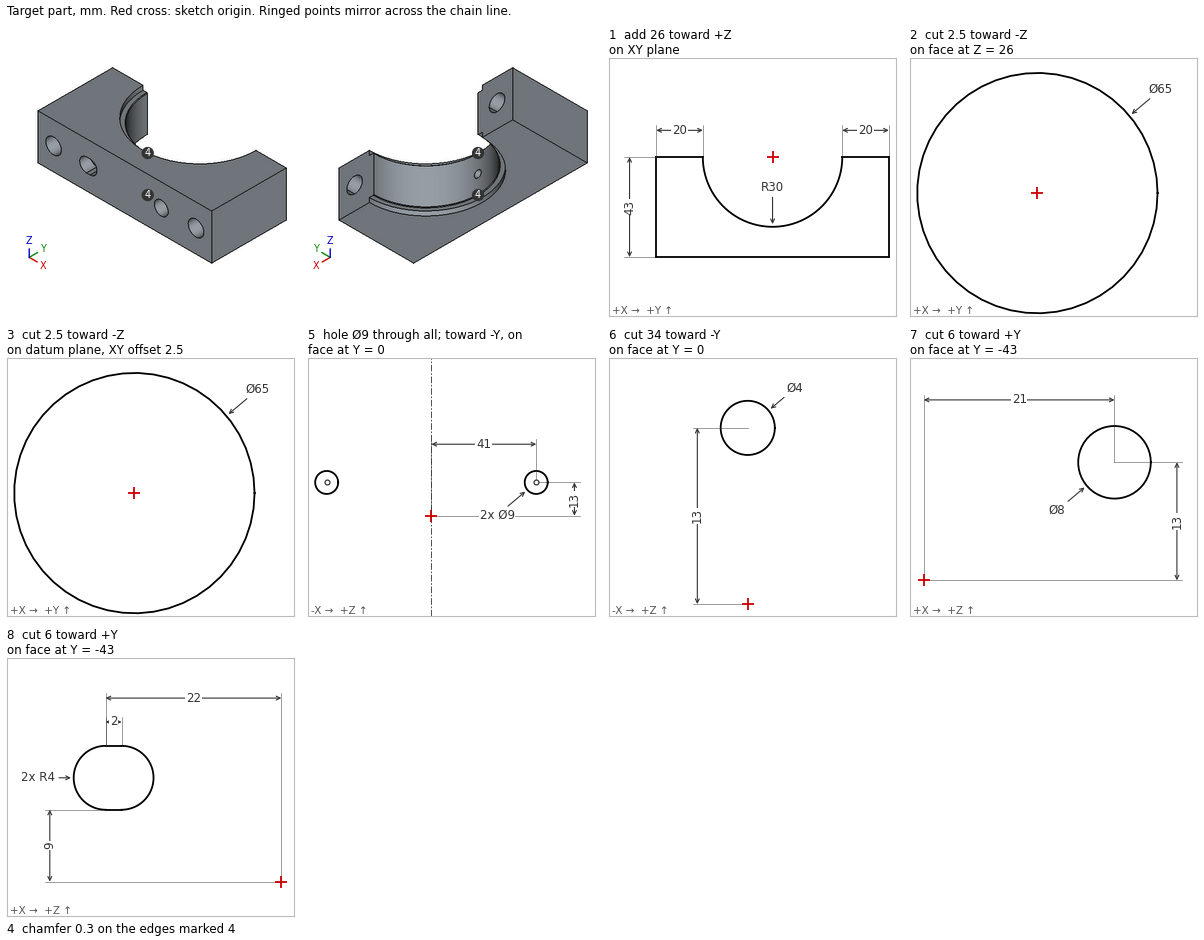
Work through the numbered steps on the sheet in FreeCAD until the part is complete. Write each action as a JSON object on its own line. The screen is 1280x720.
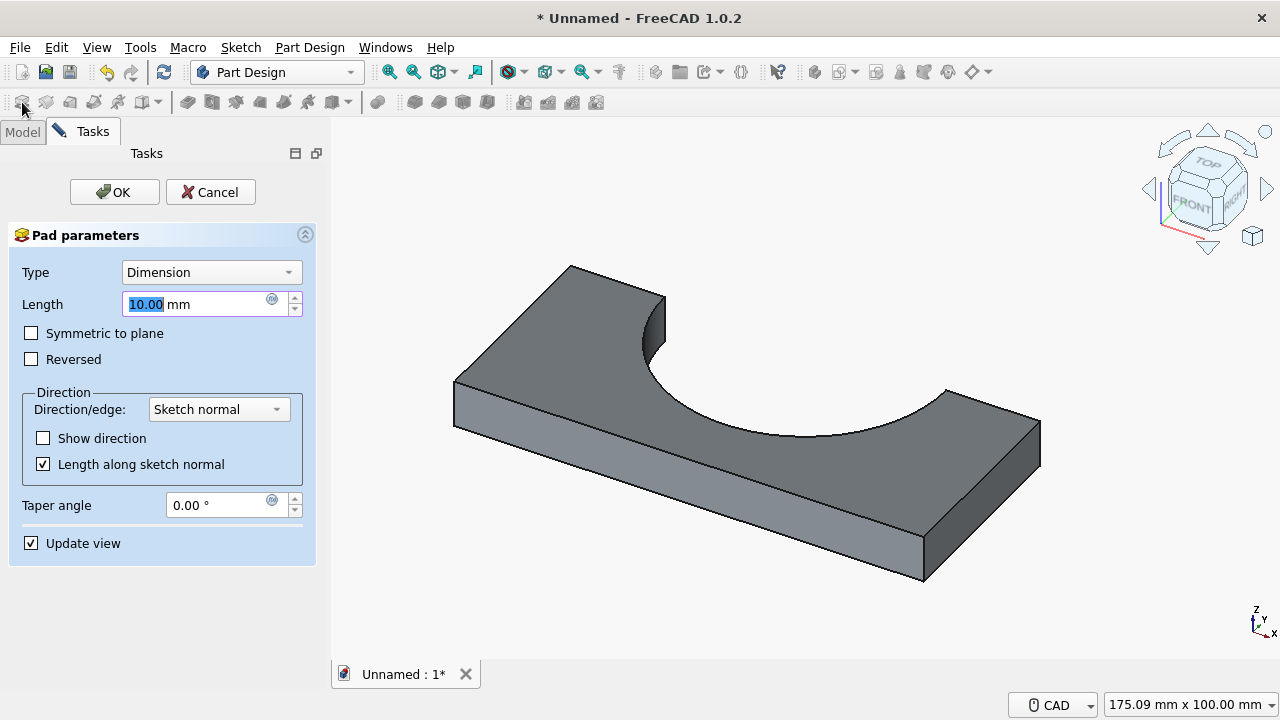
{"action": "type", "text": "26"}
{"action": "key", "text": "Tab"}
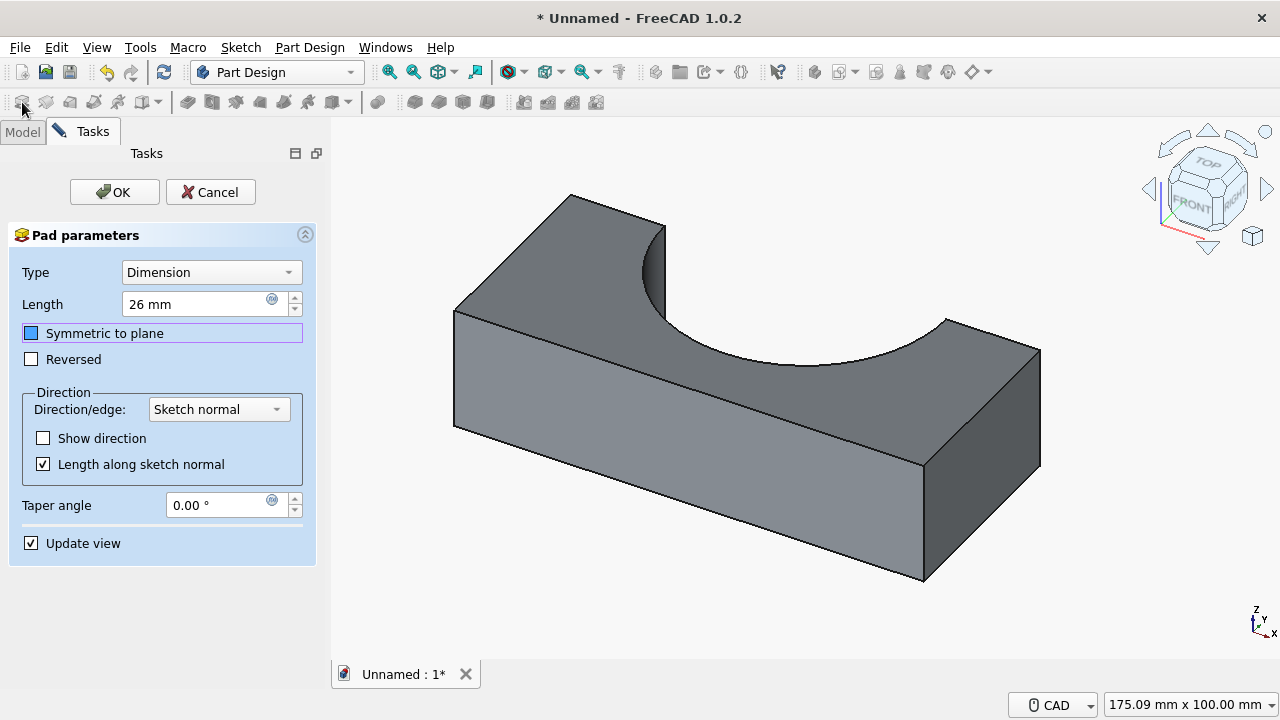
{"action": "left_click", "coordinate": [115, 192]}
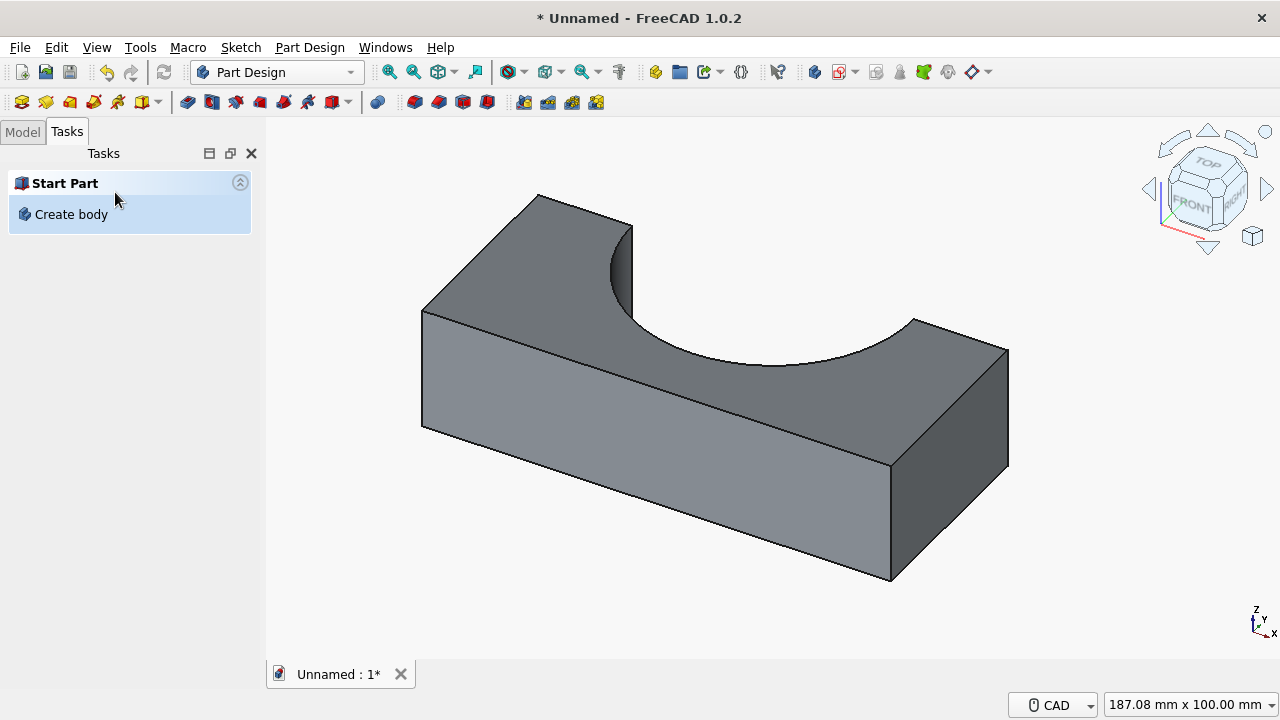
{"action": "left_click", "coordinate": [564, 302]}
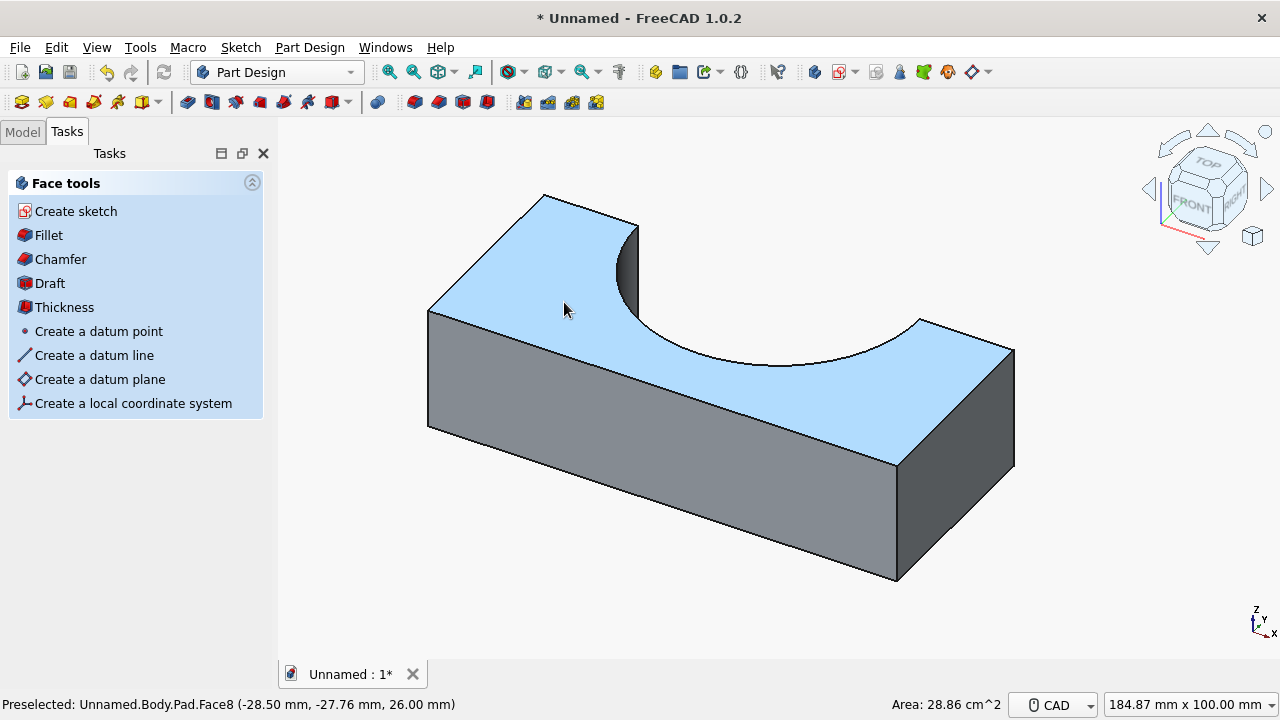
{"action": "left_click", "coordinate": [840, 72]}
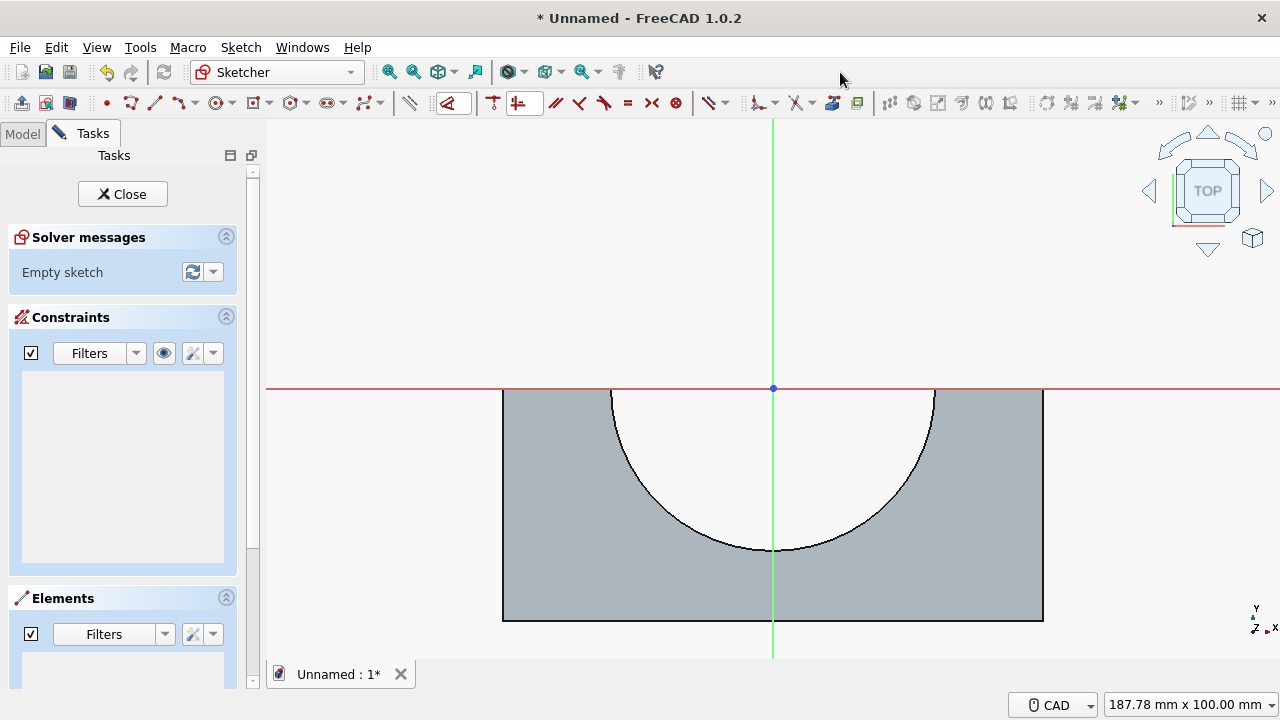
{"action": "left_click", "coordinate": [216, 104]}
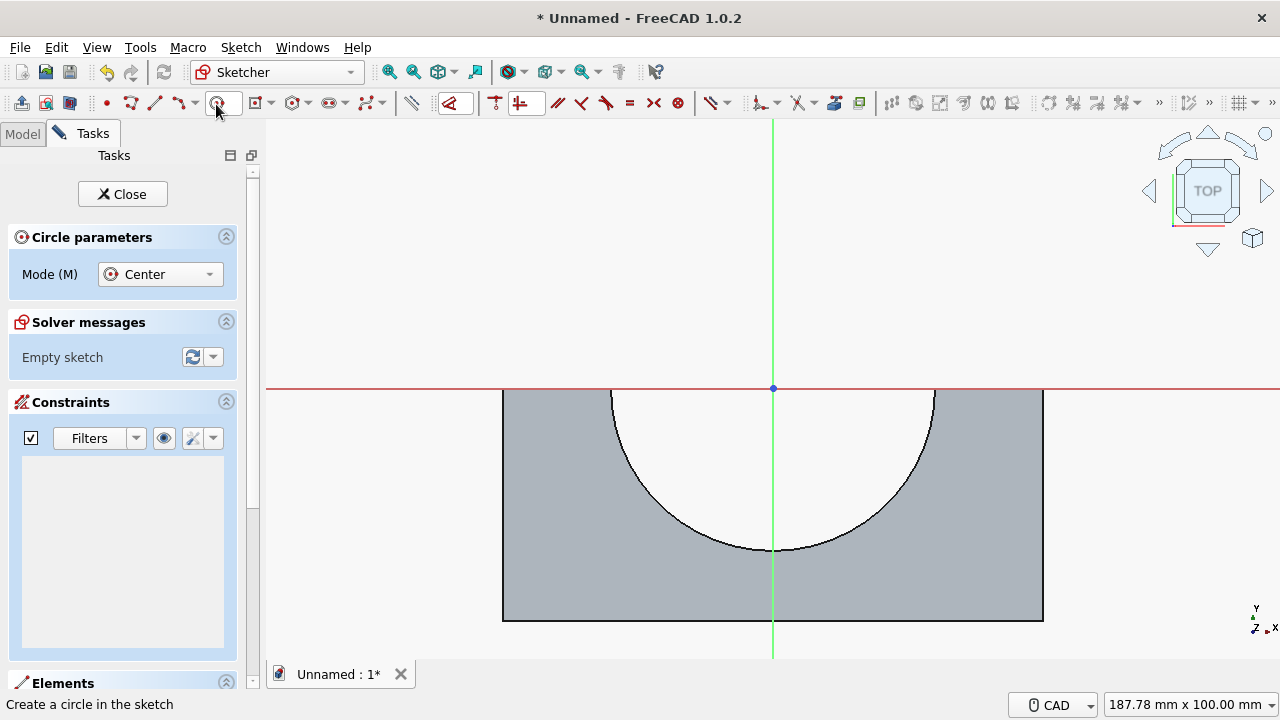
{"action": "left_click", "coordinate": [773, 389]}
{"action": "left_click", "coordinate": [897, 265]}
{"action": "key", "text": "Escape"}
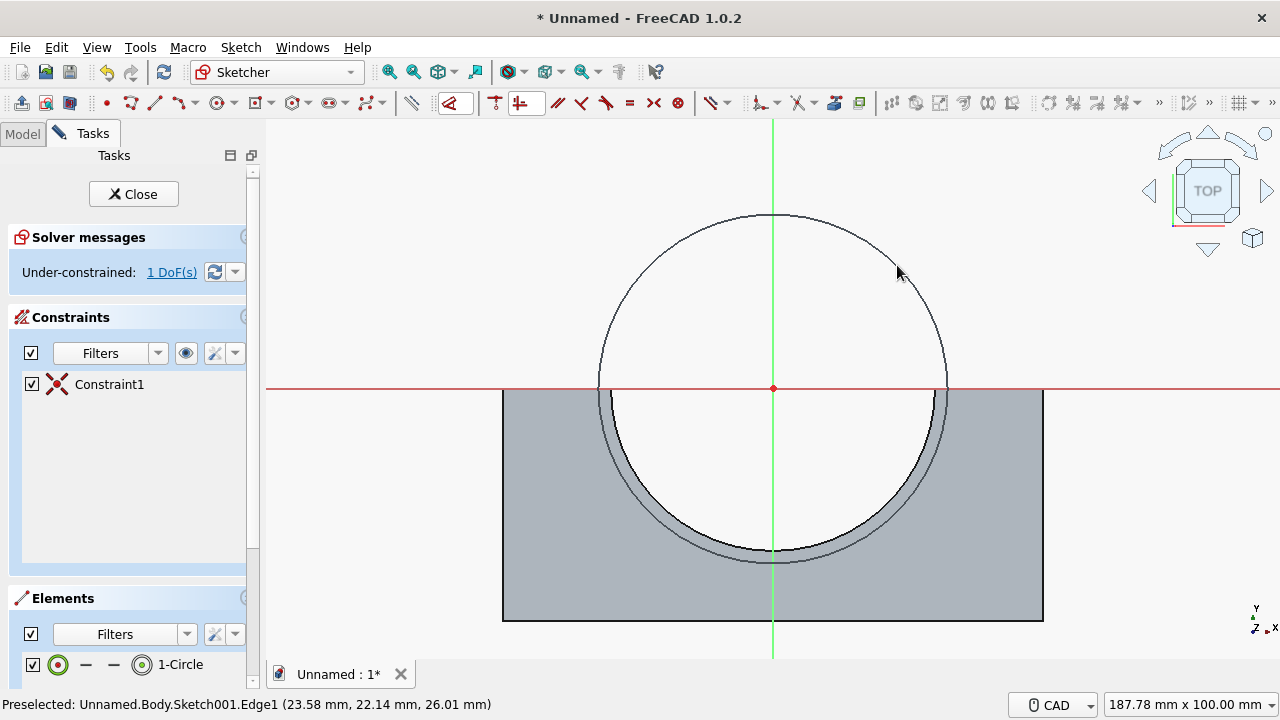
{"action": "left_click", "coordinate": [896, 265]}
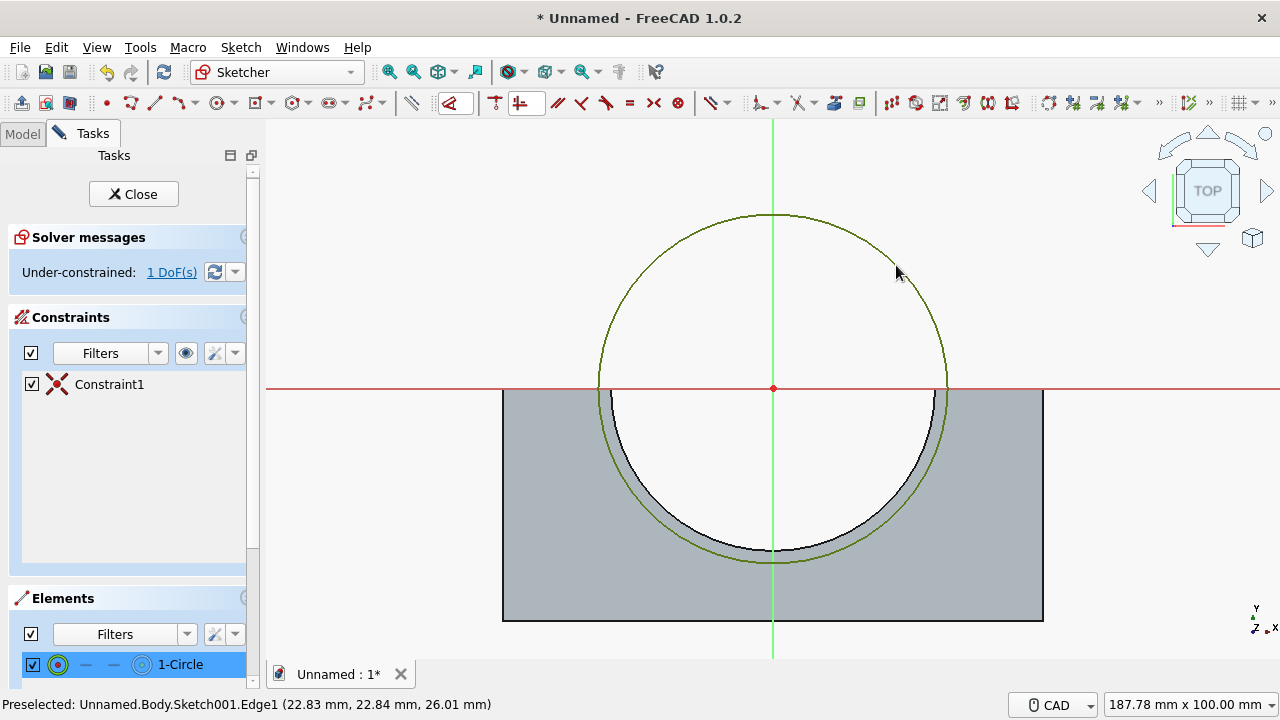
{"action": "left_click", "coordinate": [468, 104]}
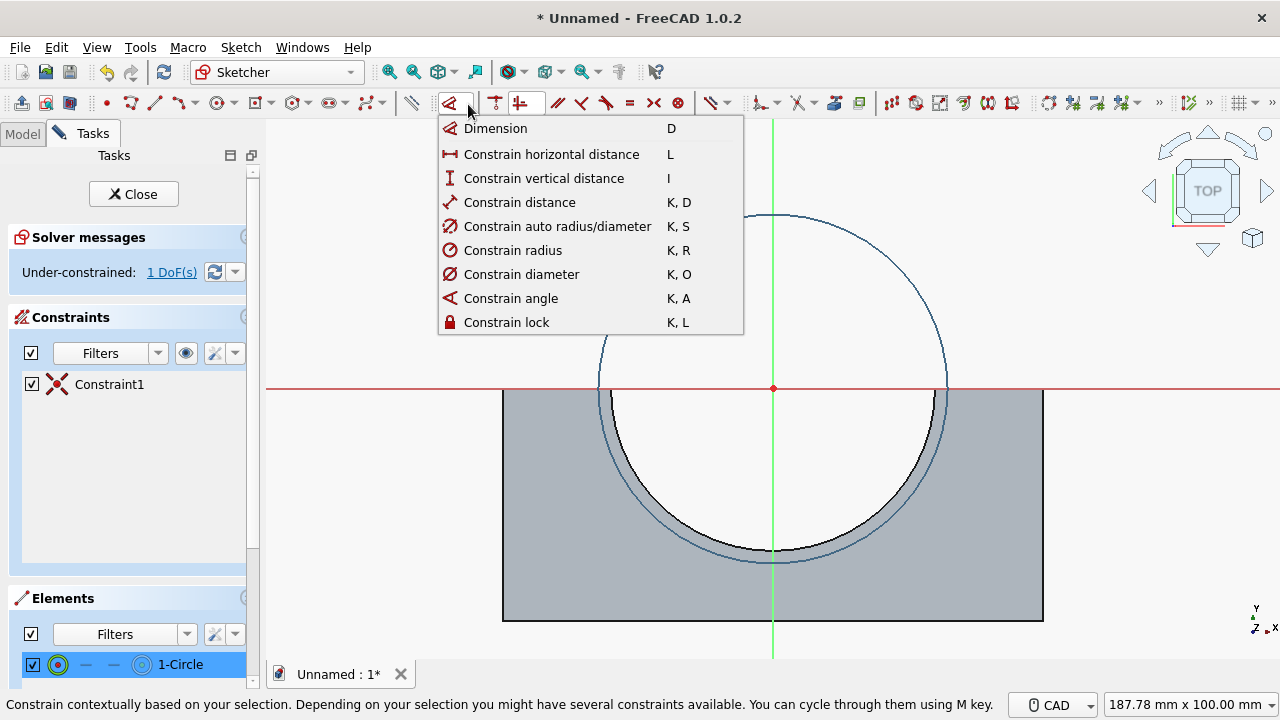
{"action": "left_click", "coordinate": [591, 274]}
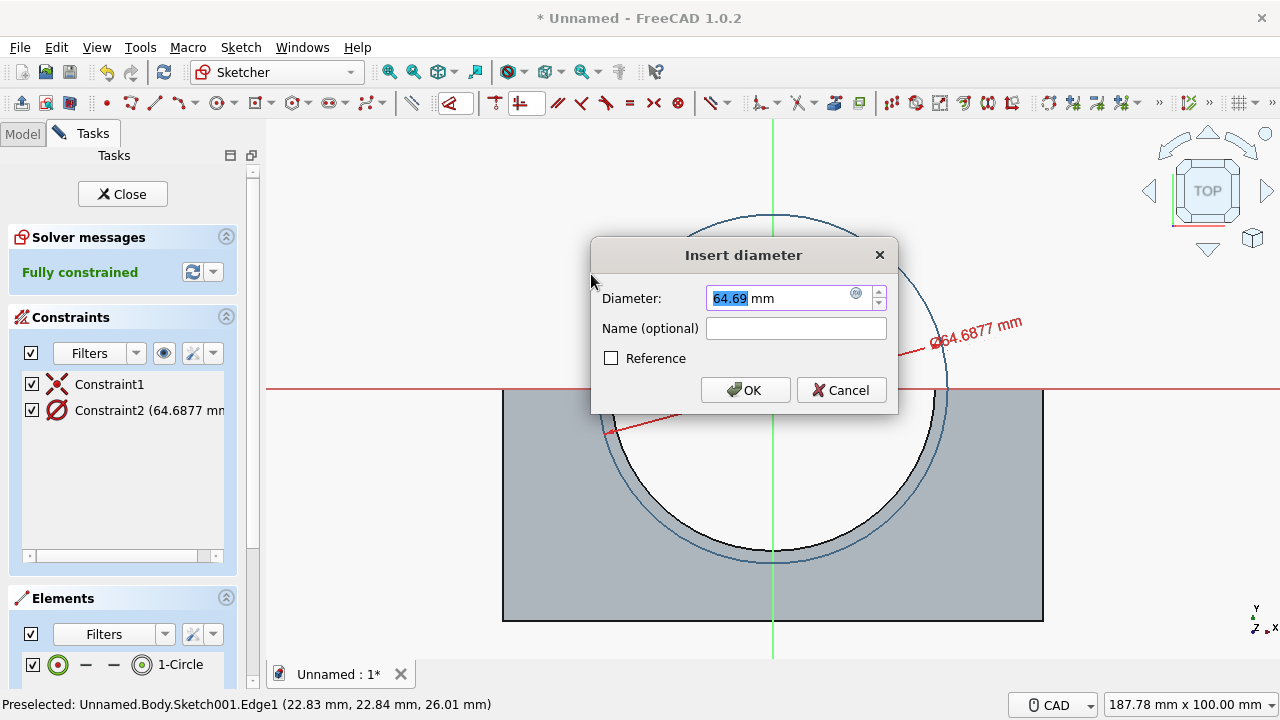
{"action": "type", "text": "65"}
{"action": "key", "text": "Return"}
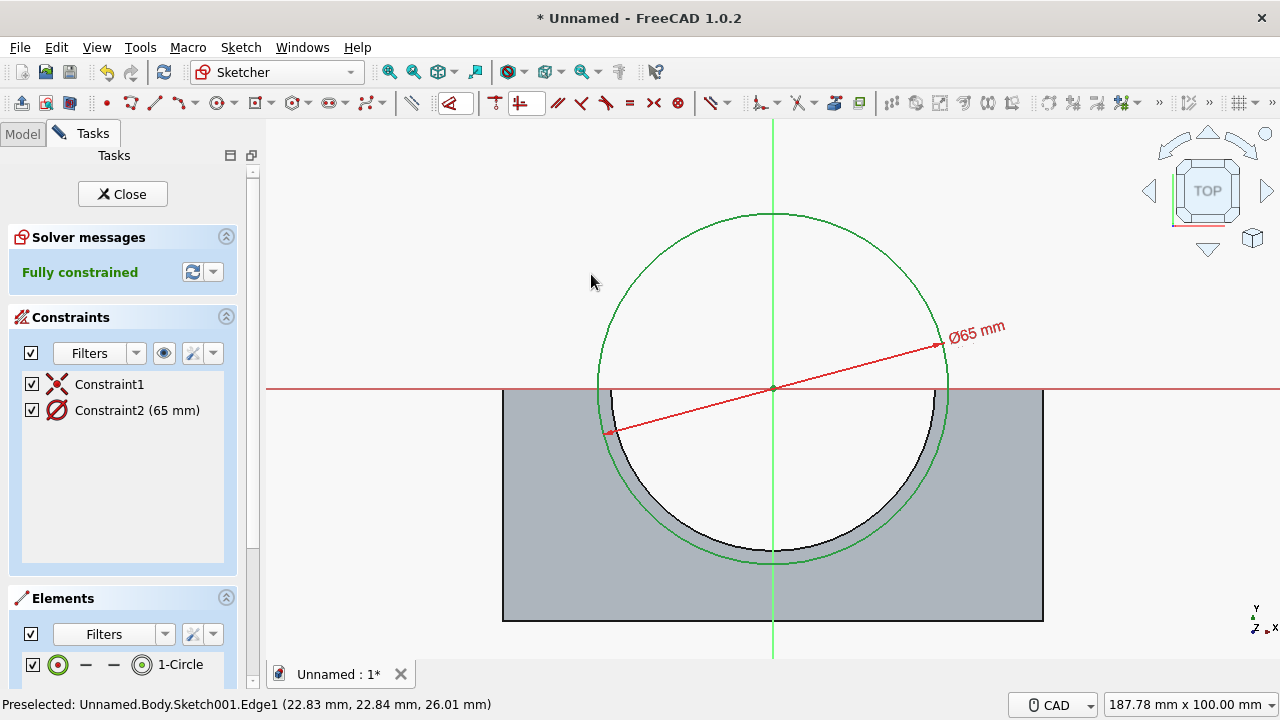
{"action": "left_click", "coordinate": [123, 194]}